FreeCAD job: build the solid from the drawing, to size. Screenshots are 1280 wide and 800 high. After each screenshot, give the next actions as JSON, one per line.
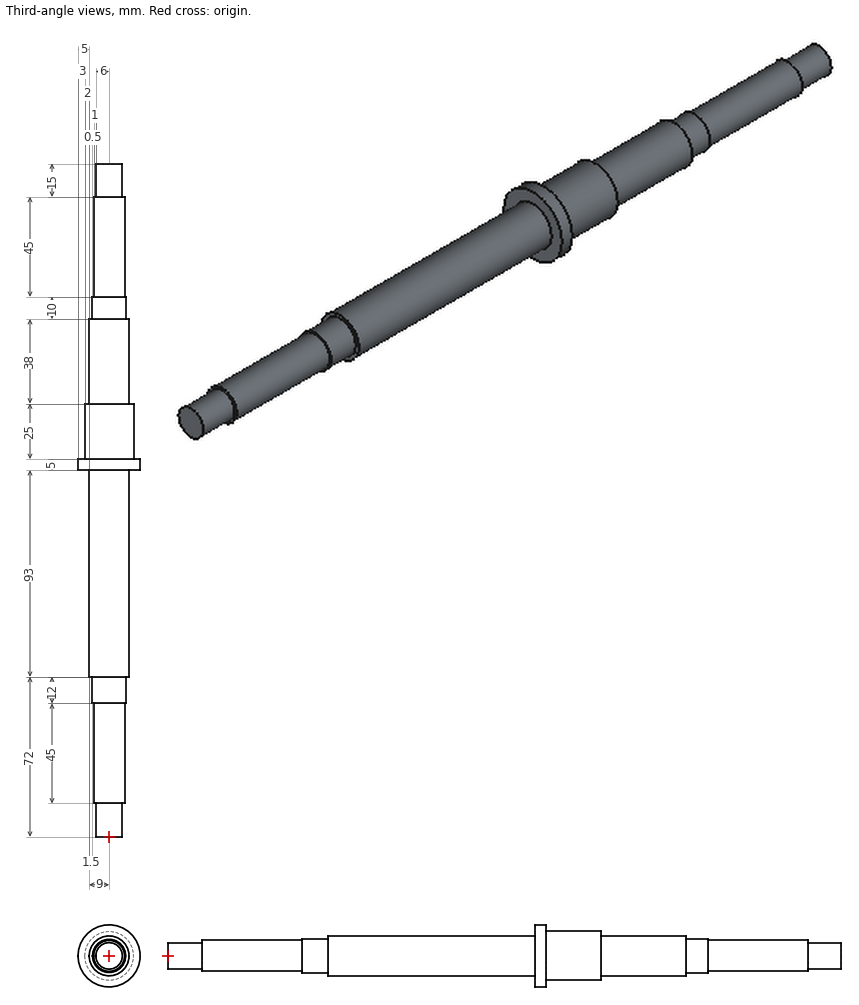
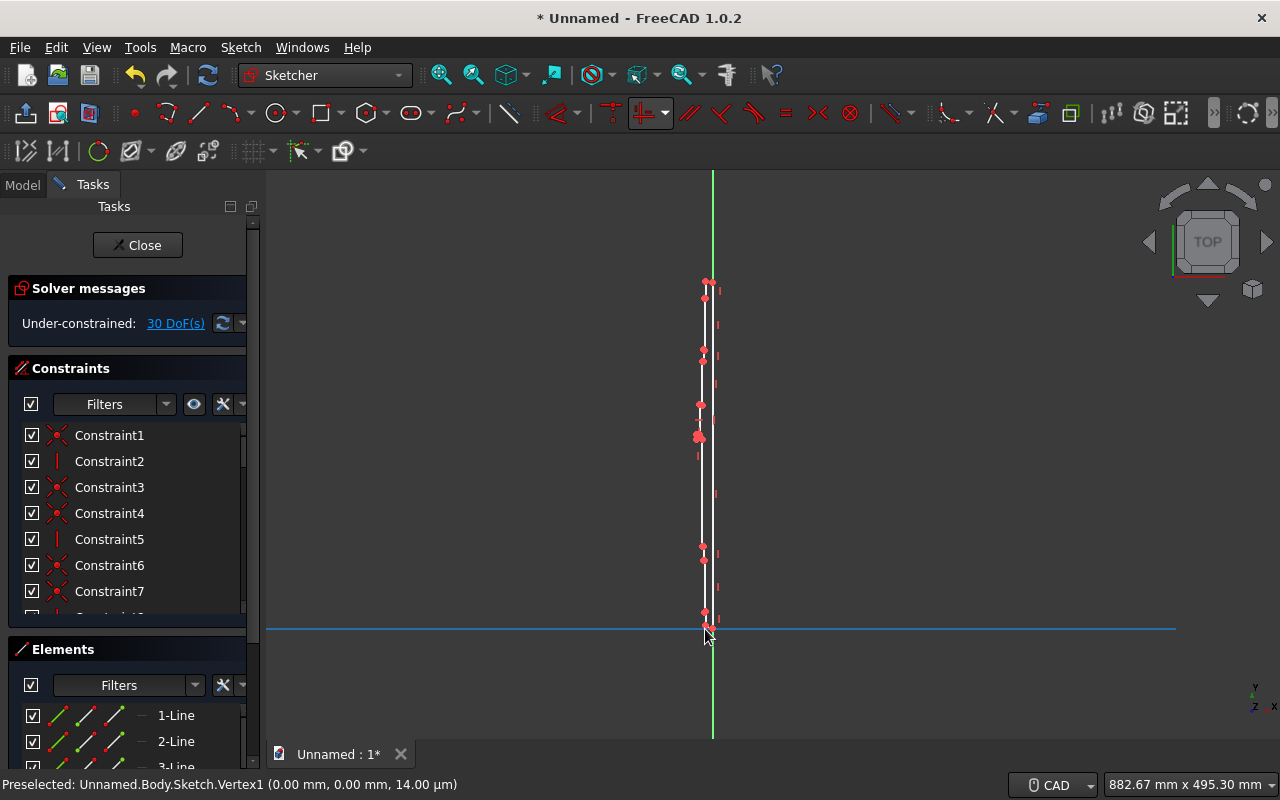
{"action": "scroll", "coordinate": [709, 282], "scroll_direction": "up", "scroll_amount": 8}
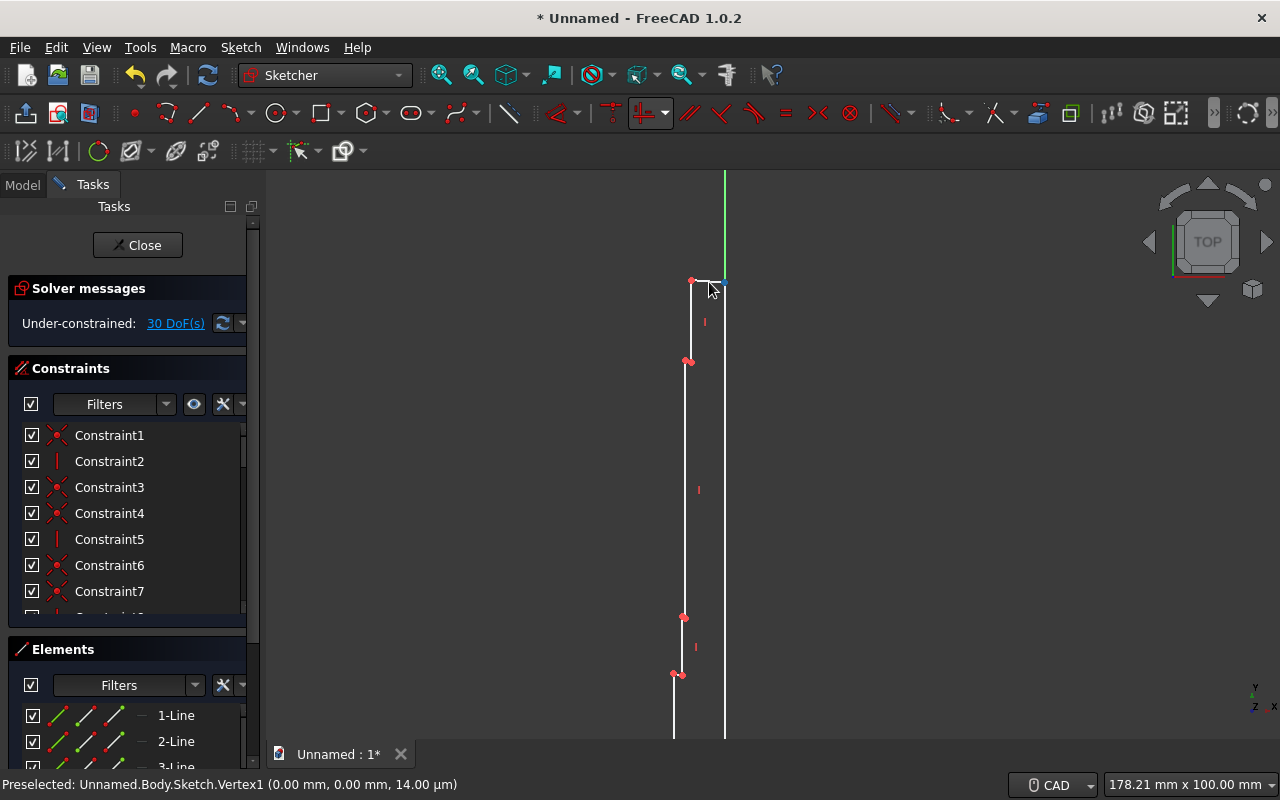
{"action": "left_click", "coordinate": [708, 281]}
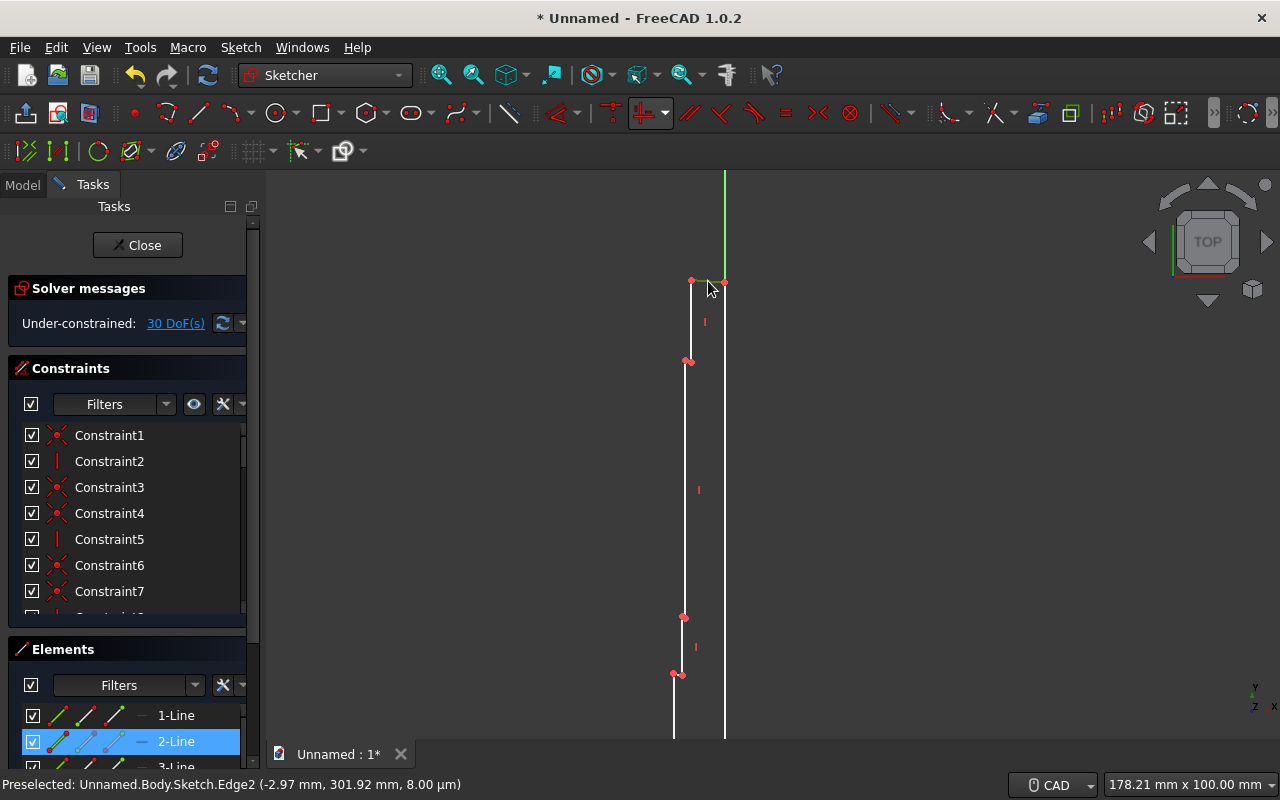
{"action": "left_click", "coordinate": [668, 114]}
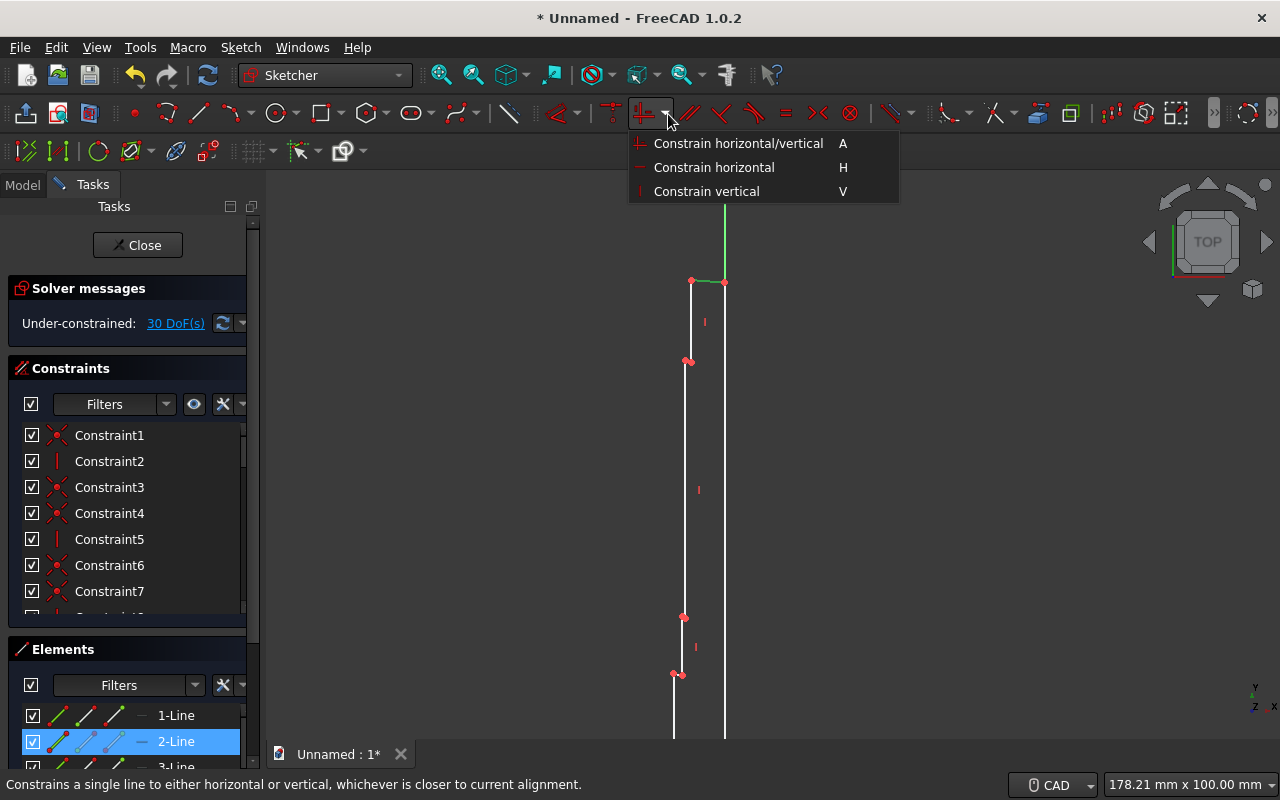
{"action": "left_click", "coordinate": [764, 167]}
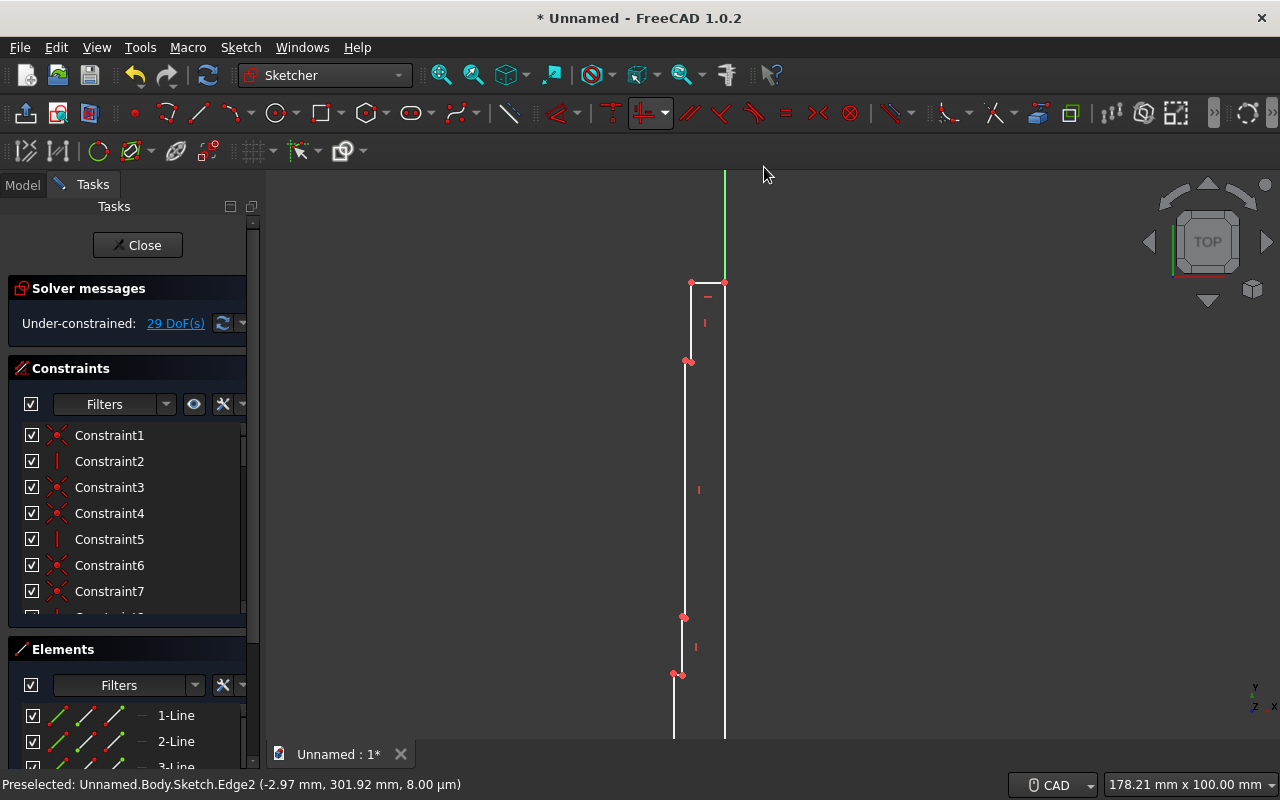
{"action": "scroll", "coordinate": [688, 361], "scroll_direction": "up", "scroll_amount": 6}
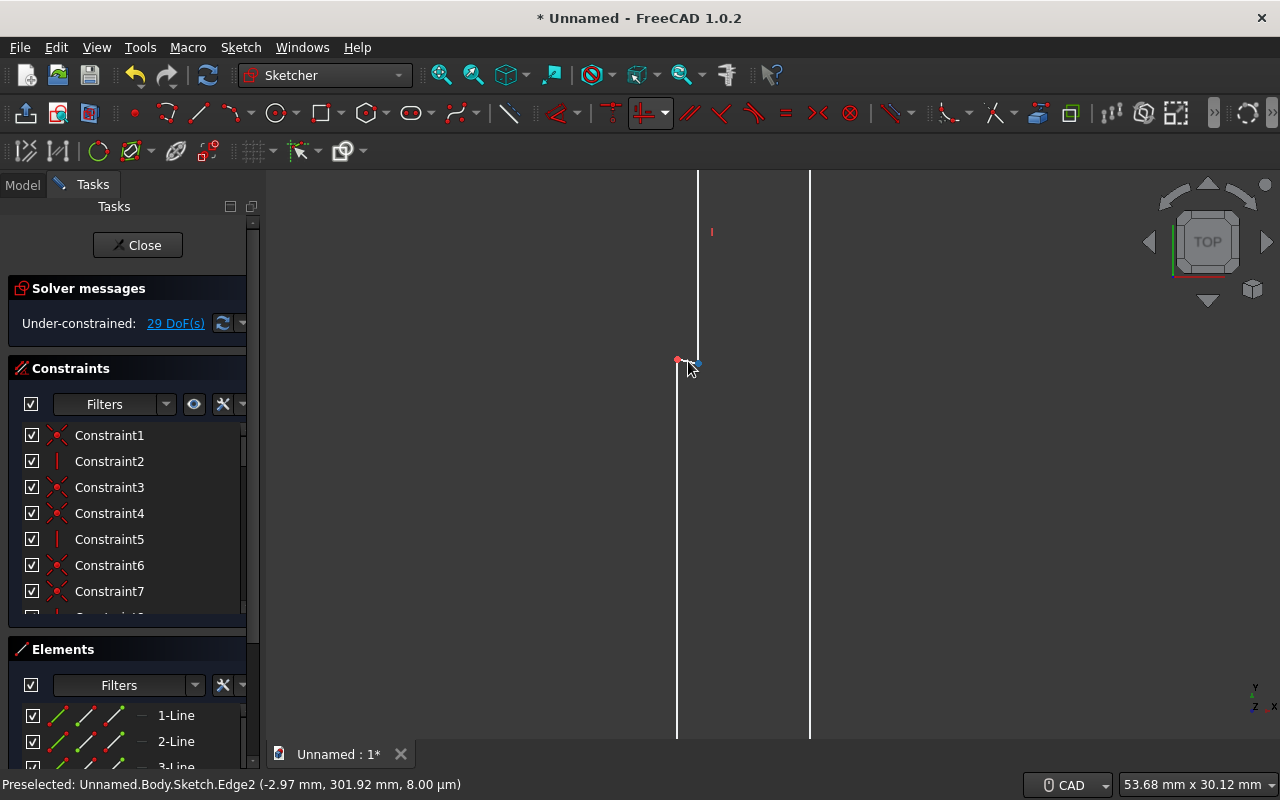
{"action": "left_click", "coordinate": [688, 361]}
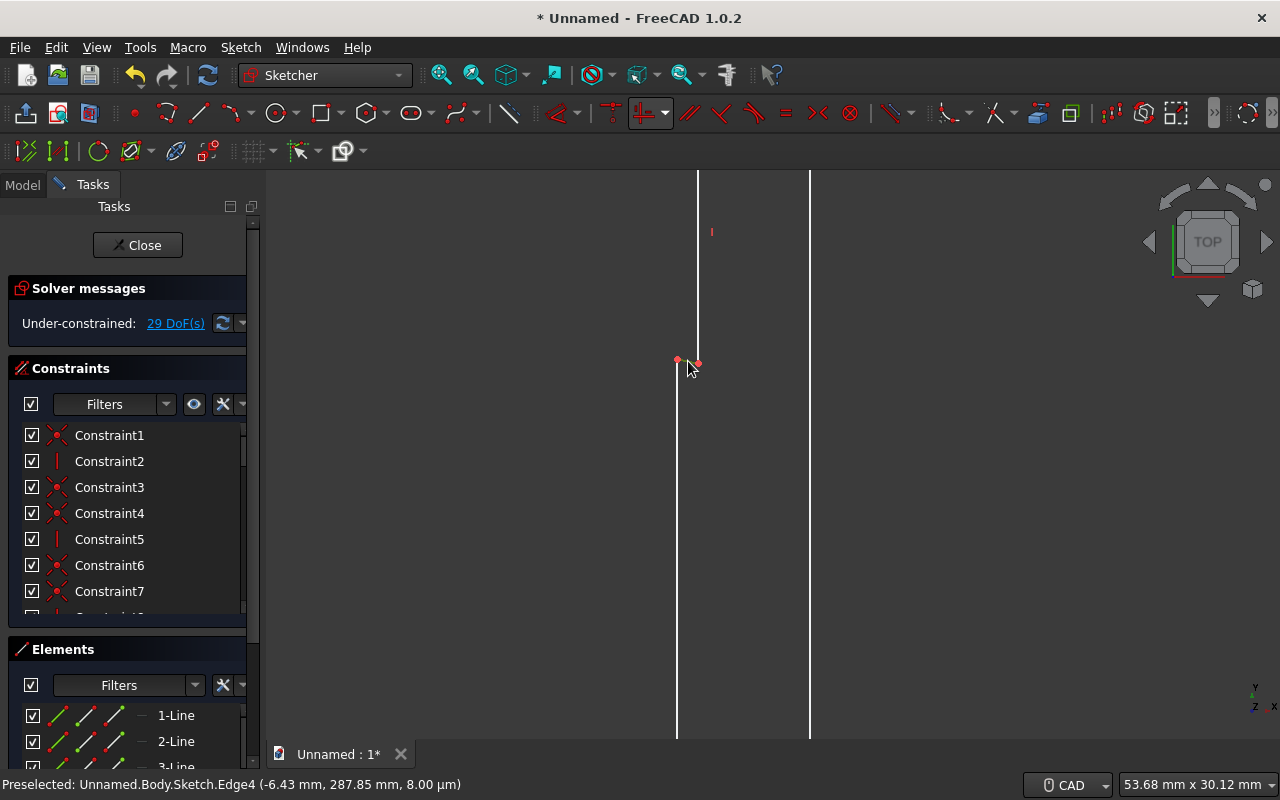
{"action": "key", "text": "h"}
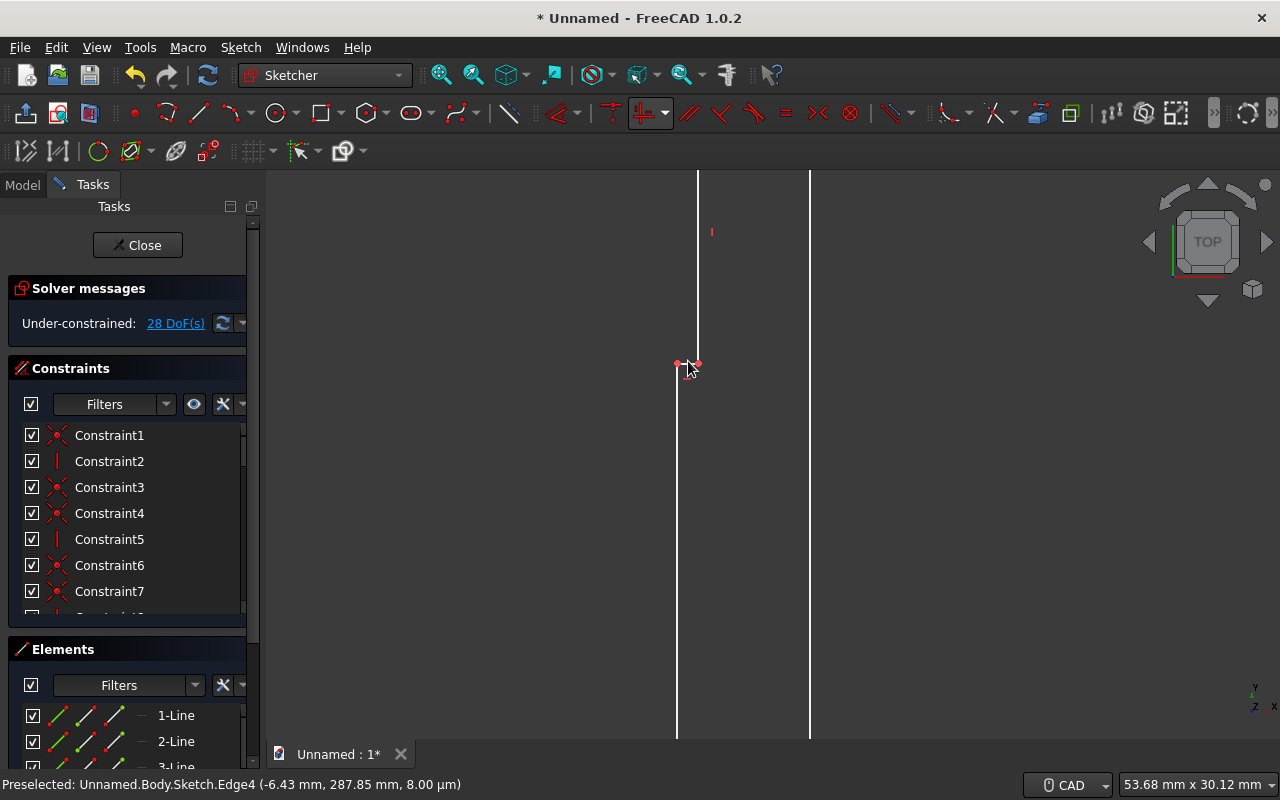
{"action": "scroll", "coordinate": [706, 294], "scroll_direction": "down", "scroll_amount": 14}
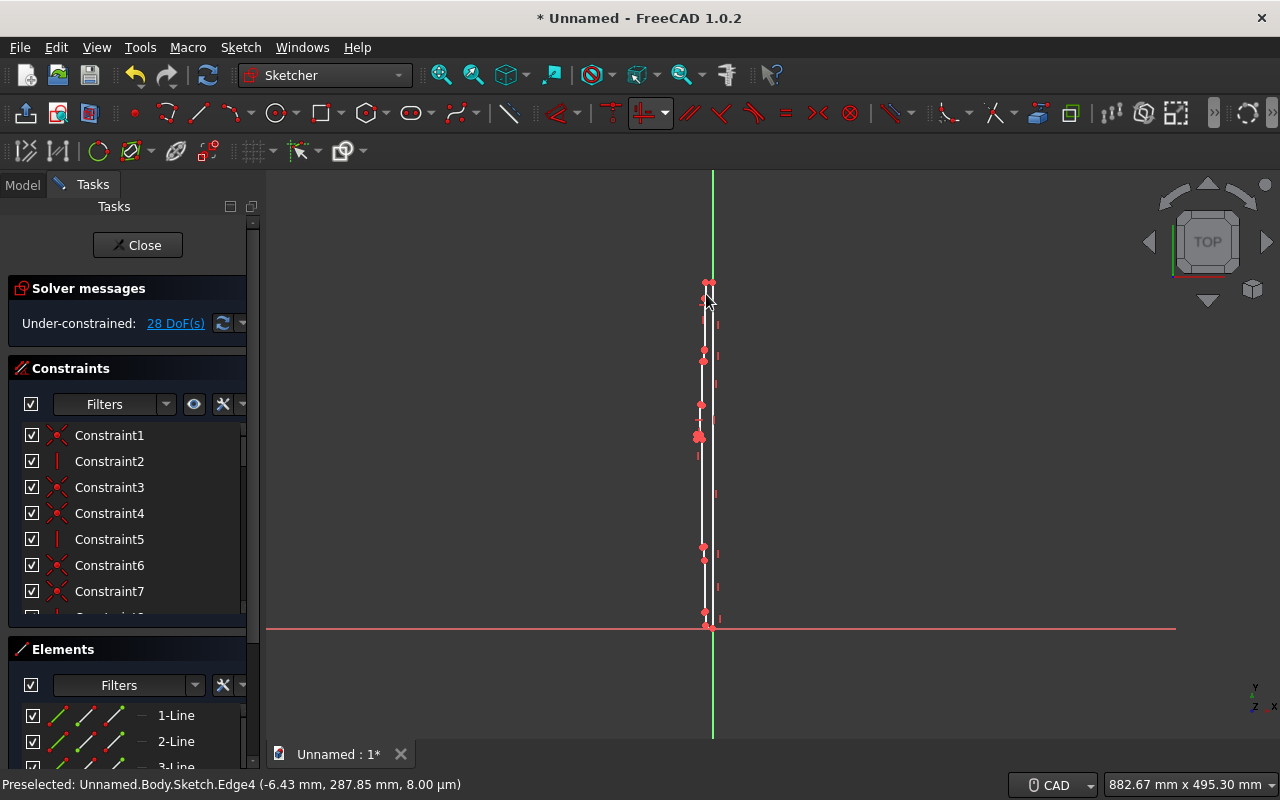
{"action": "scroll", "coordinate": [704, 350], "scroll_direction": "up", "scroll_amount": 14}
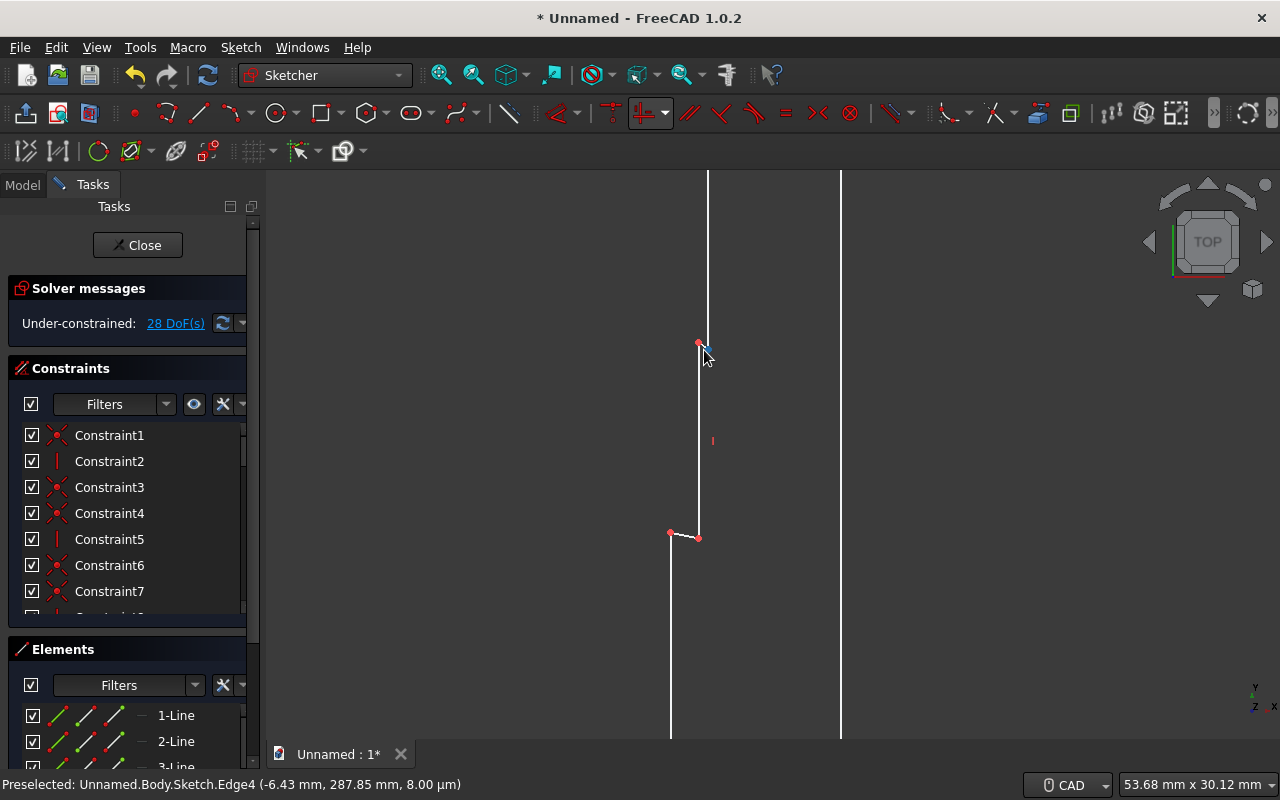
{"action": "left_click", "coordinate": [703, 346]}